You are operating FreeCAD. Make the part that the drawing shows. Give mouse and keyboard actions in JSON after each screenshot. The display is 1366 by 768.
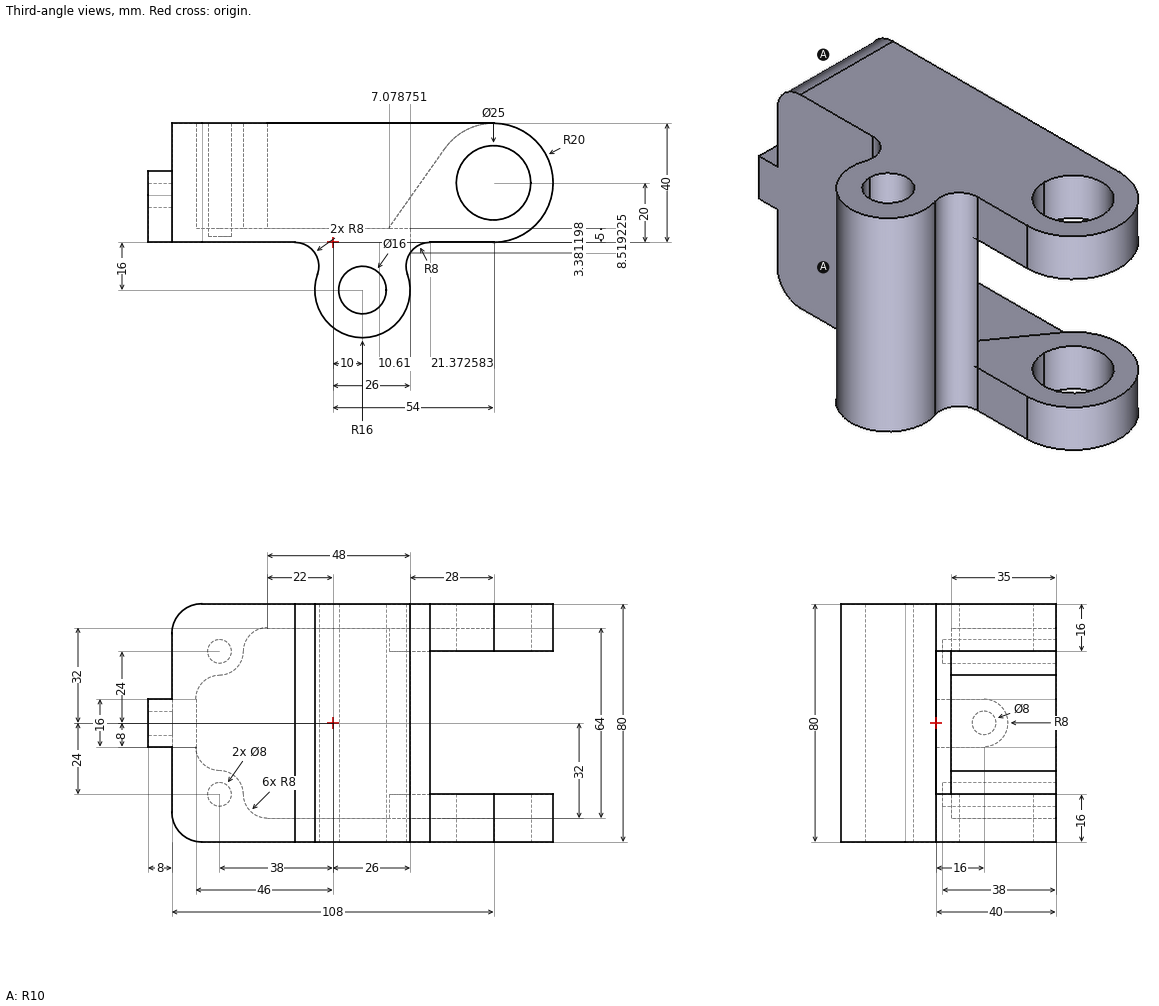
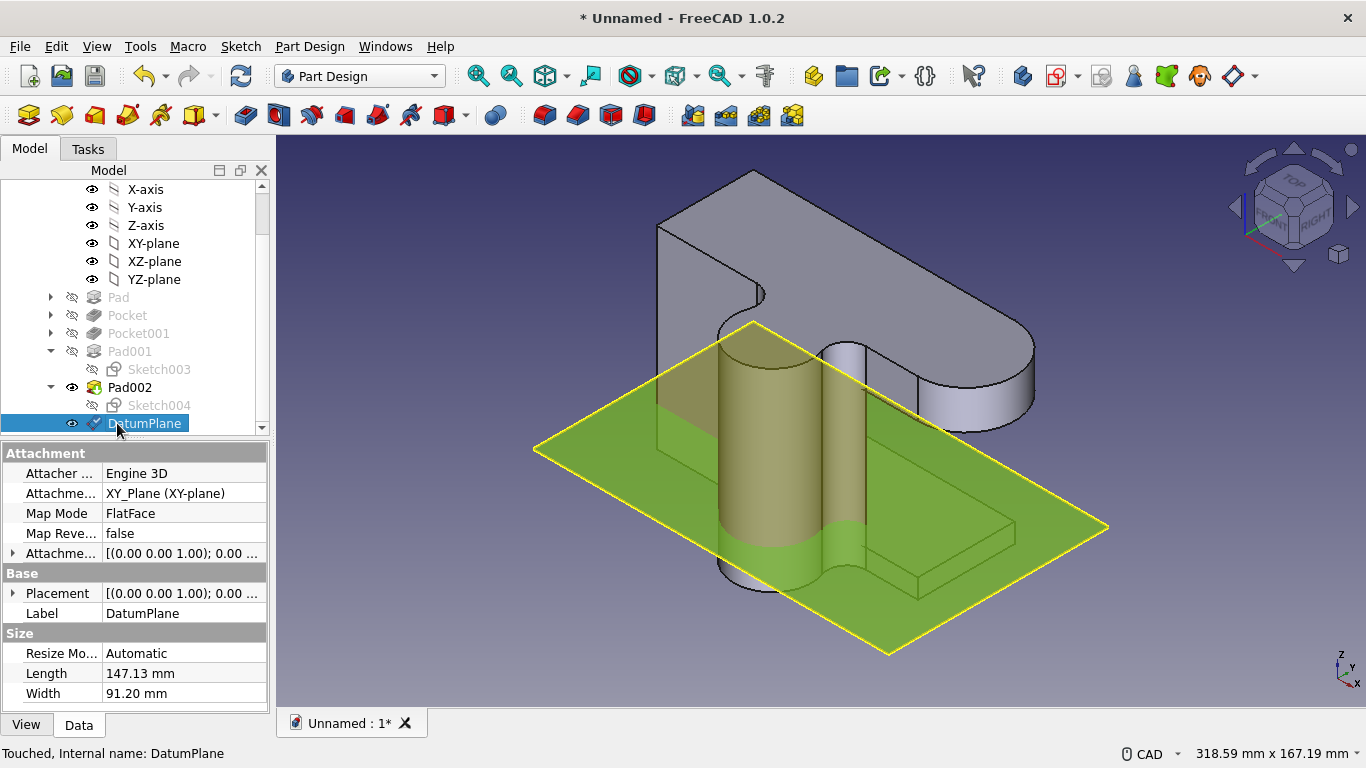
{"action": "left_click", "coordinate": [1056, 76]}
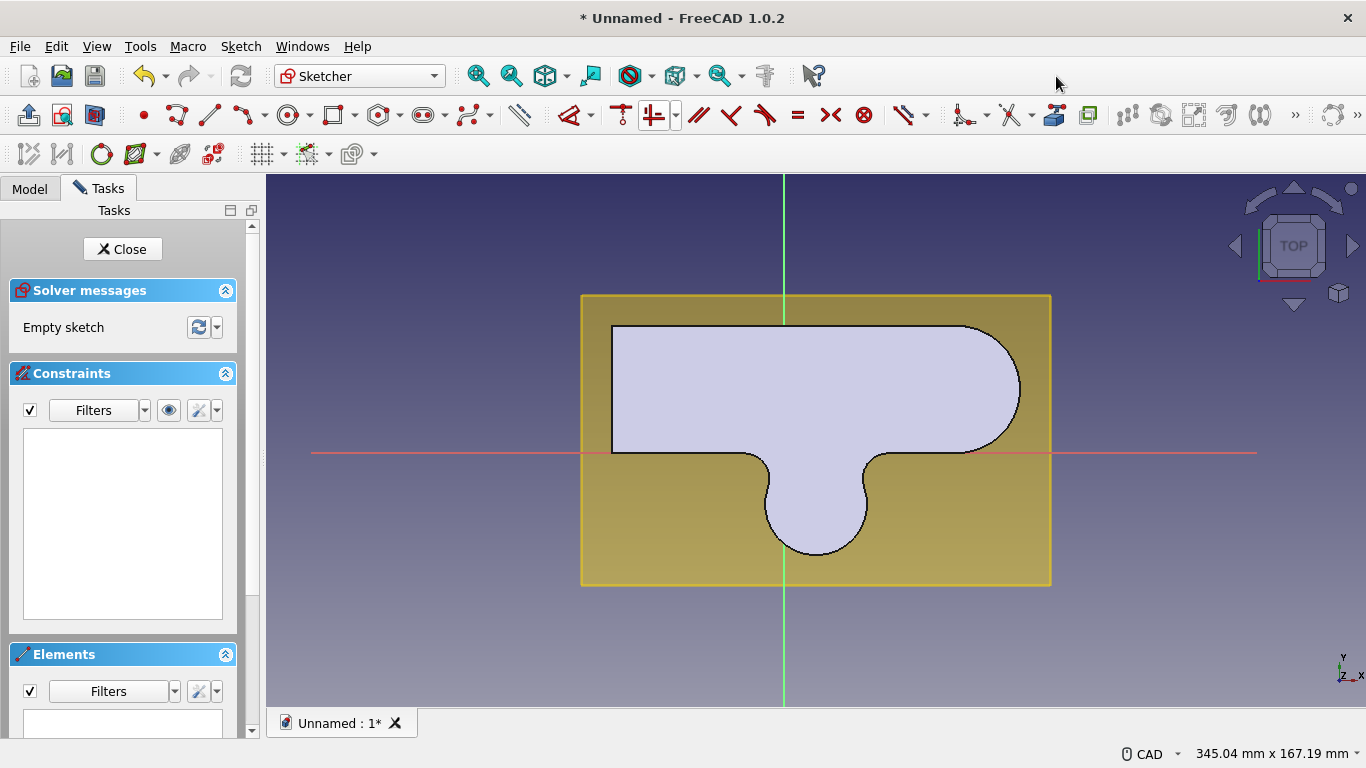
{"action": "left_click", "coordinate": [95, 116]}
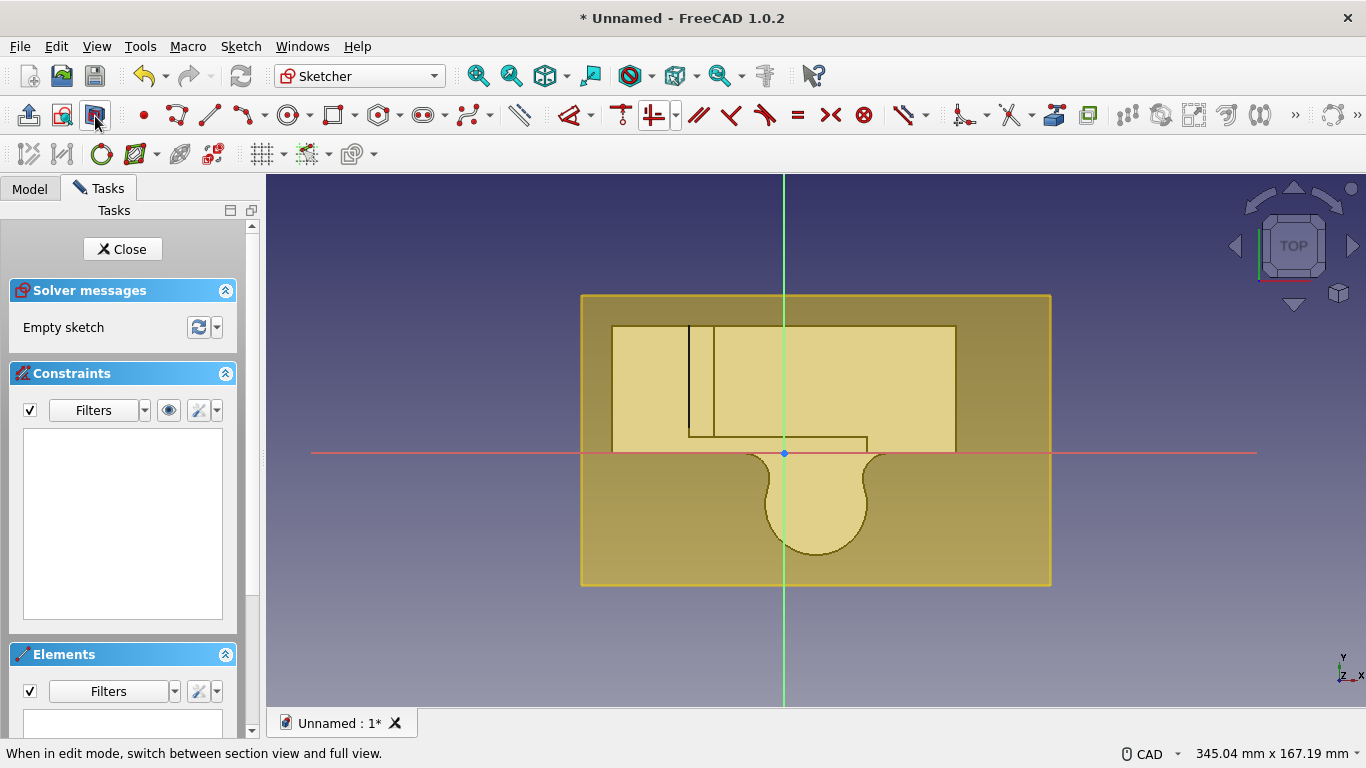
{"action": "scroll", "coordinate": [987, 390], "scroll_direction": "up", "scroll_amount": 5}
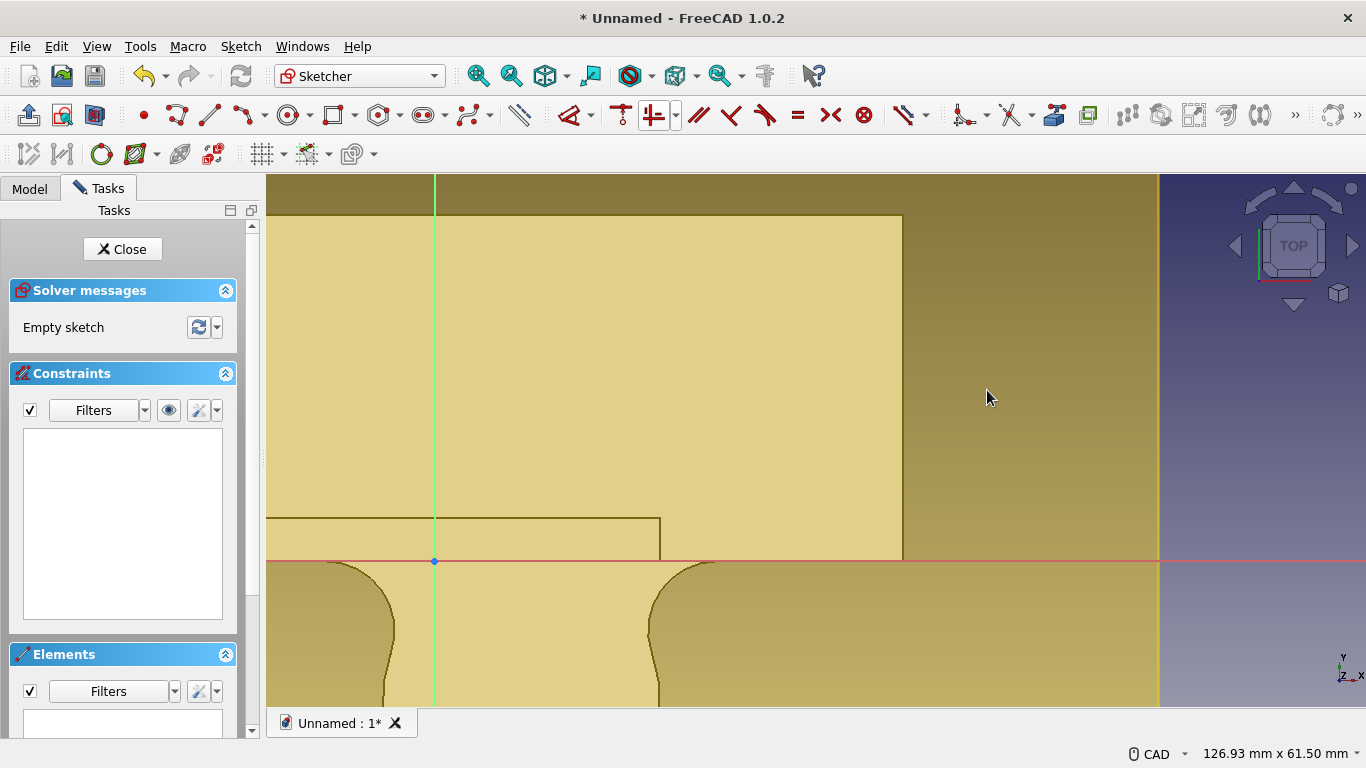
{"action": "key", "text": "g l"}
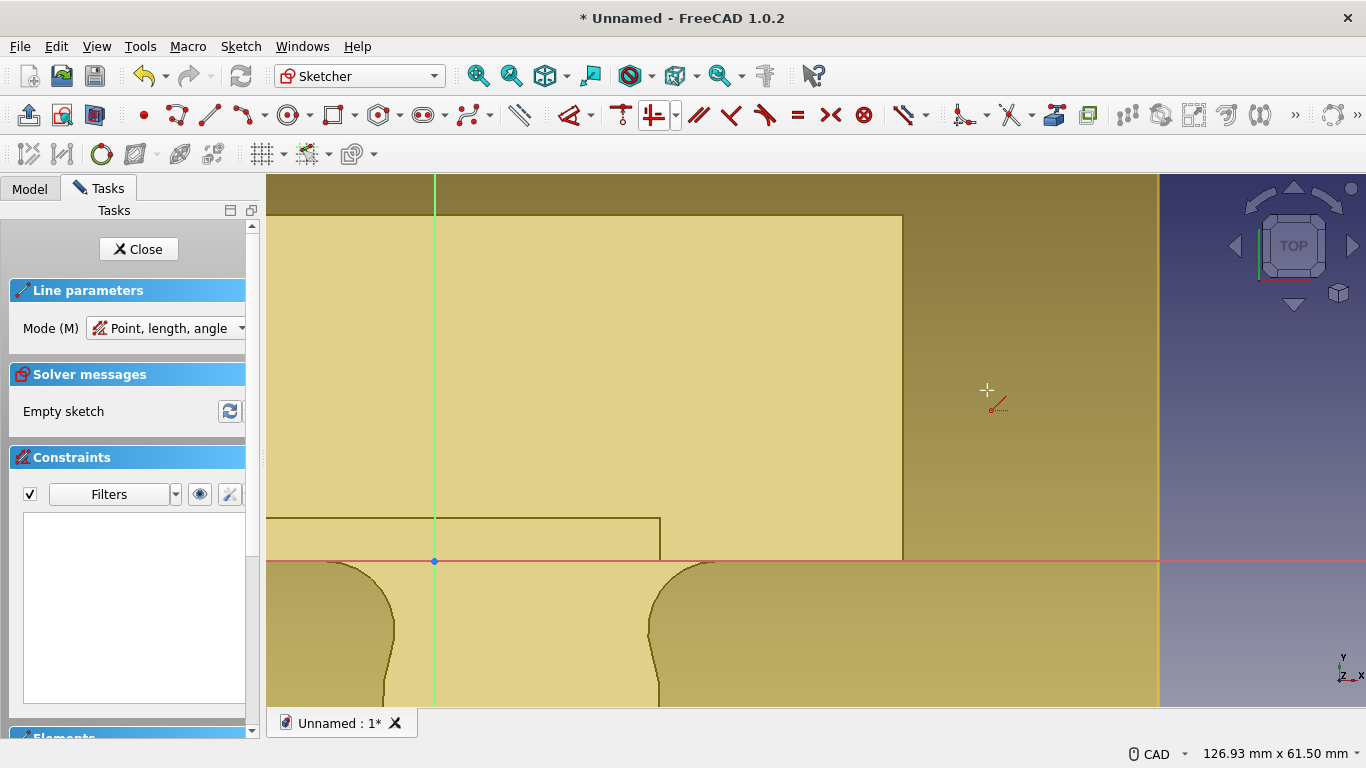
{"action": "left_click", "coordinate": [903, 561]}
{"action": "left_click", "coordinate": [717, 552]}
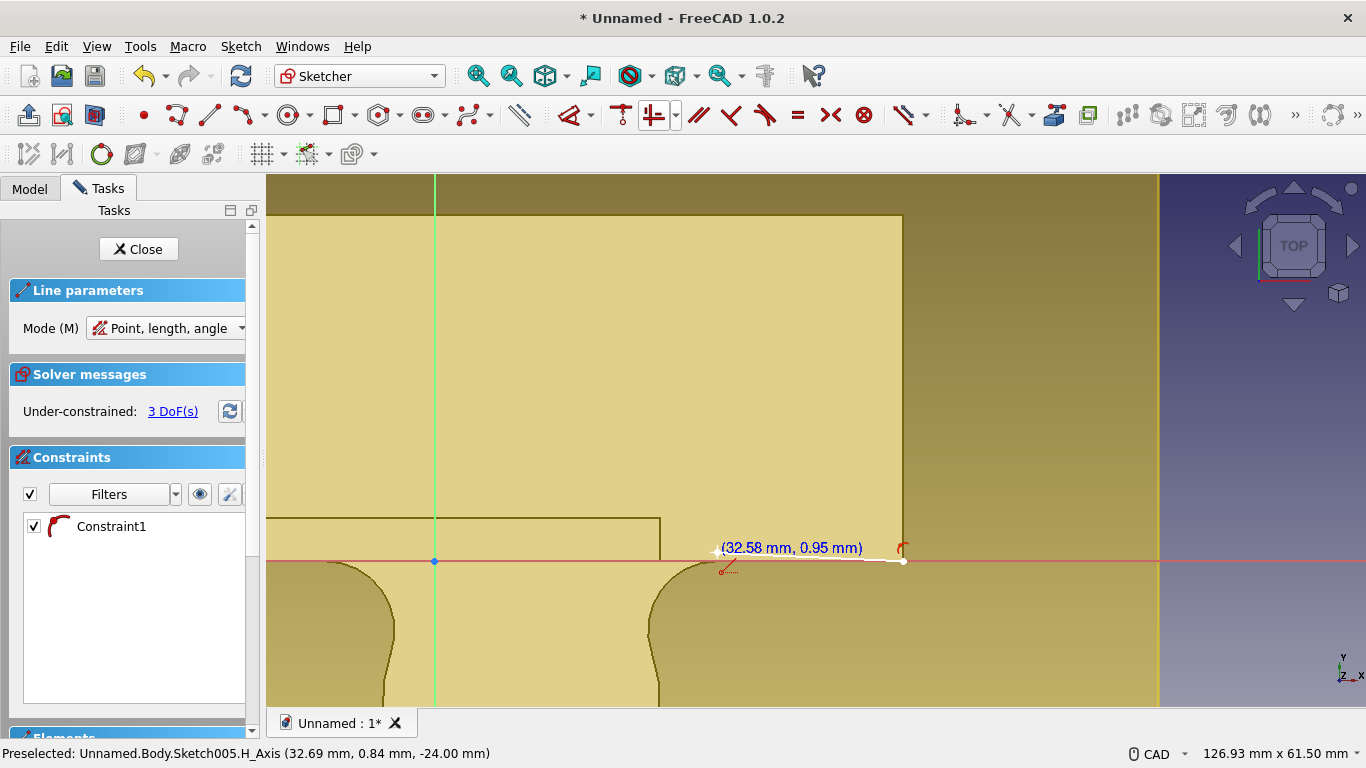
{"action": "key", "text": "g m"}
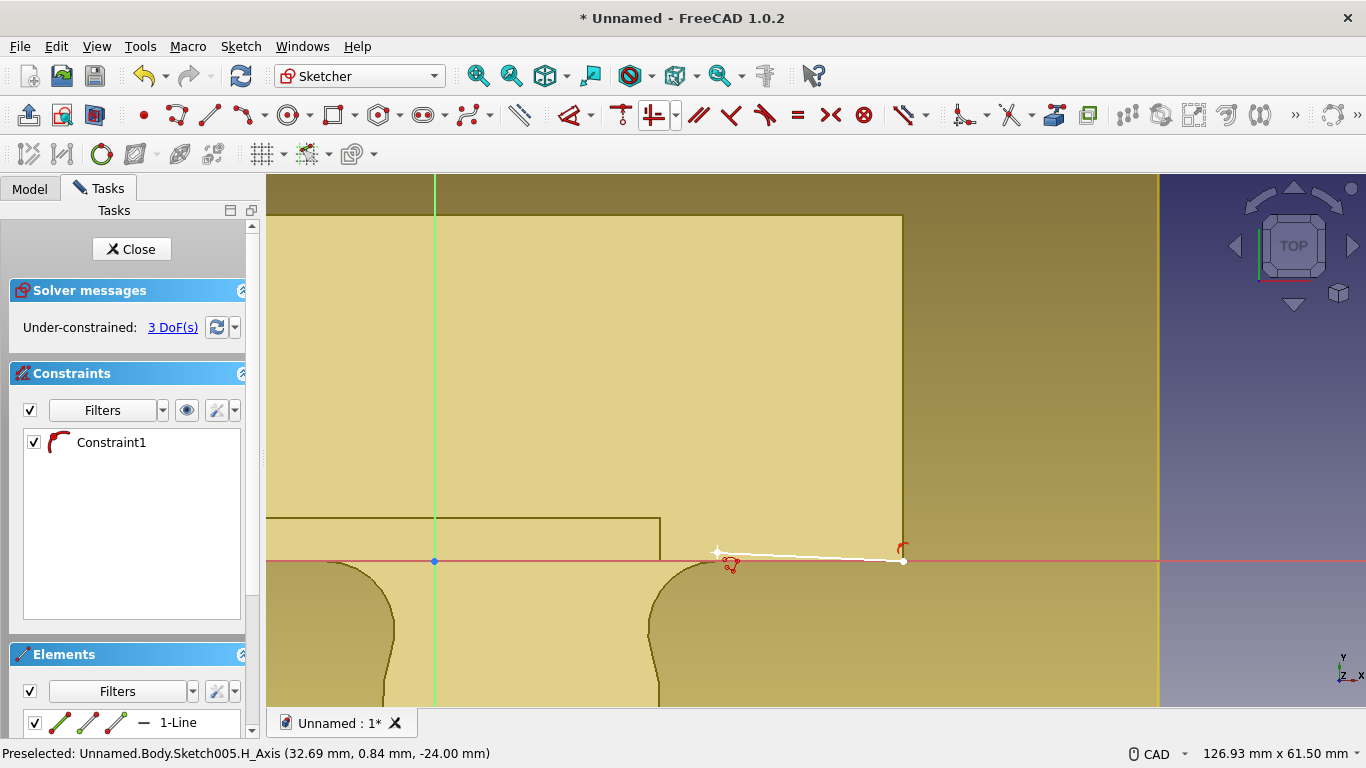
{"action": "left_click", "coordinate": [660, 592]}
{"action": "left_click", "coordinate": [660, 518]}
{"action": "left_click", "coordinate": [599, 518]}
{"action": "left_click", "coordinate": [761, 288]}
{"action": "right_click", "coordinate": [761, 288]}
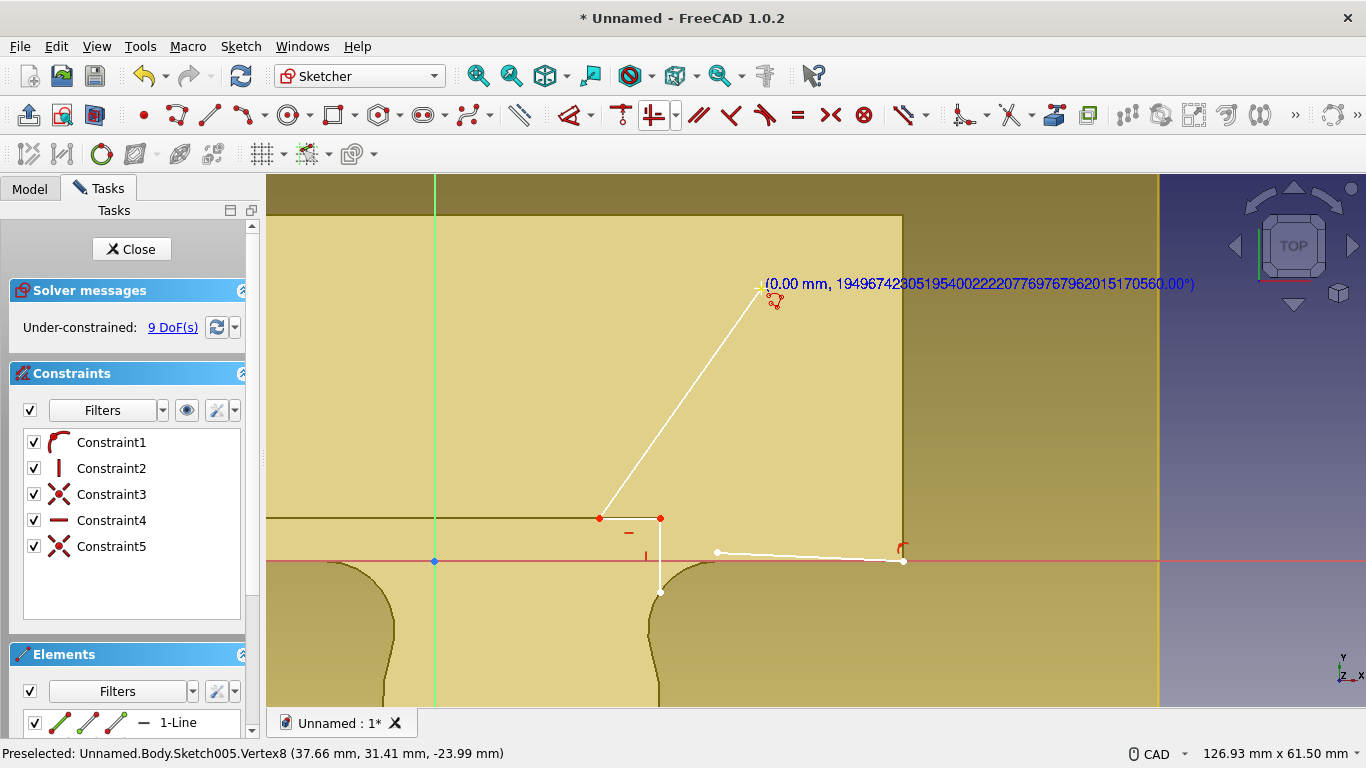
{"action": "key", "text": "g 3 a"}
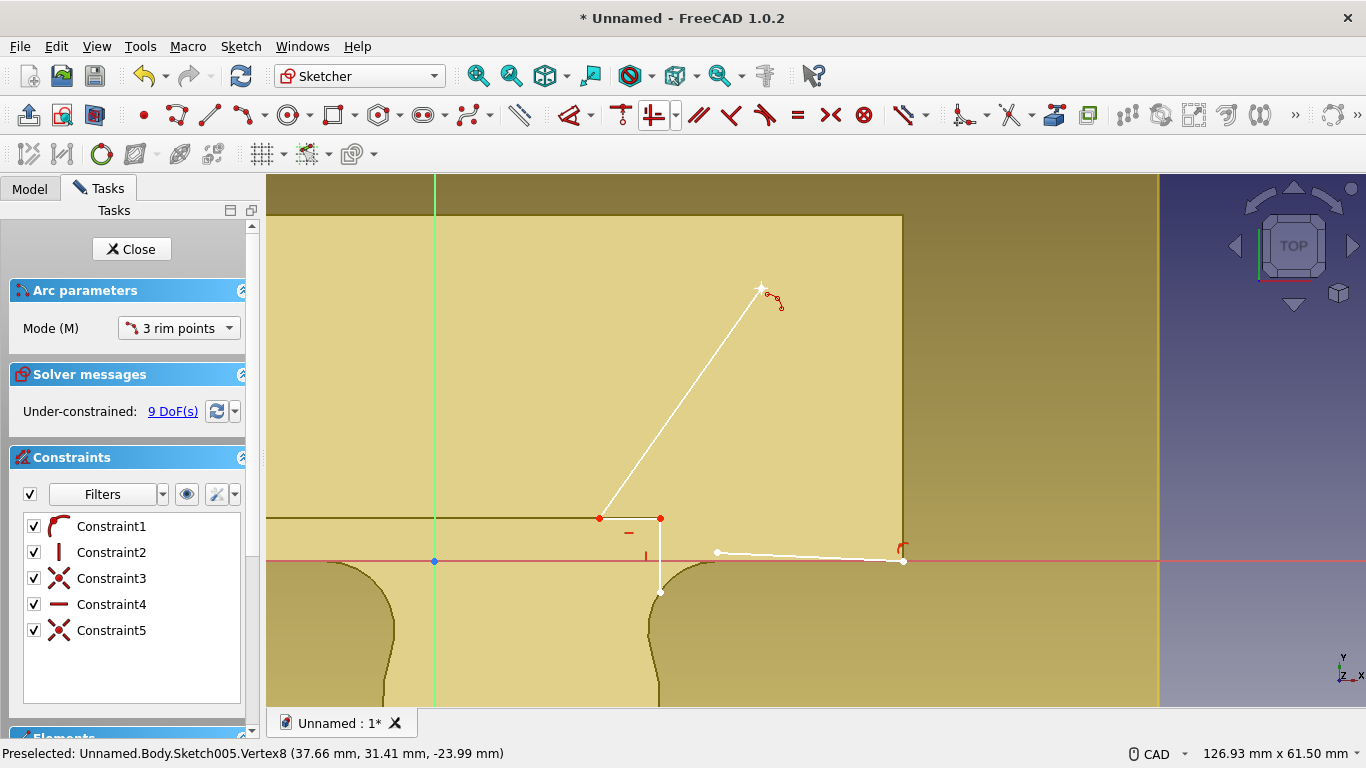
{"action": "left_click", "coordinate": [717, 553]}
{"action": "left_click", "coordinate": [660, 593]}